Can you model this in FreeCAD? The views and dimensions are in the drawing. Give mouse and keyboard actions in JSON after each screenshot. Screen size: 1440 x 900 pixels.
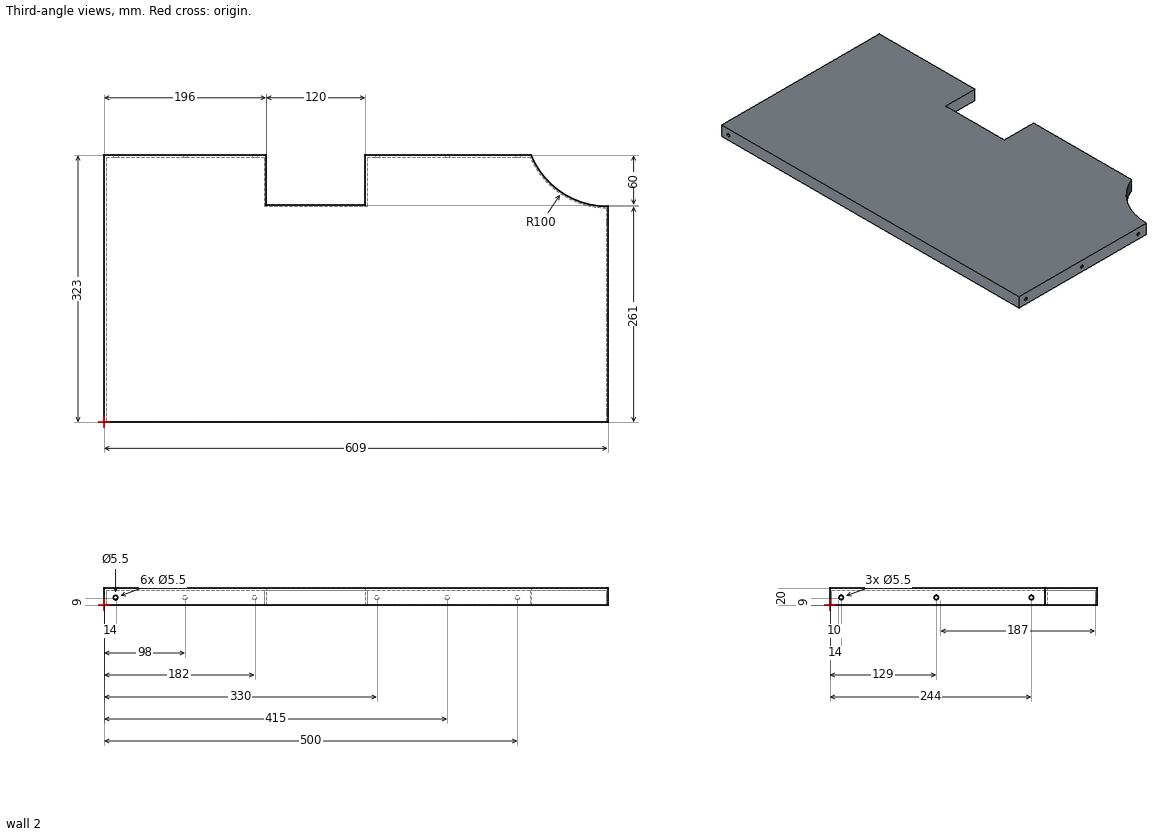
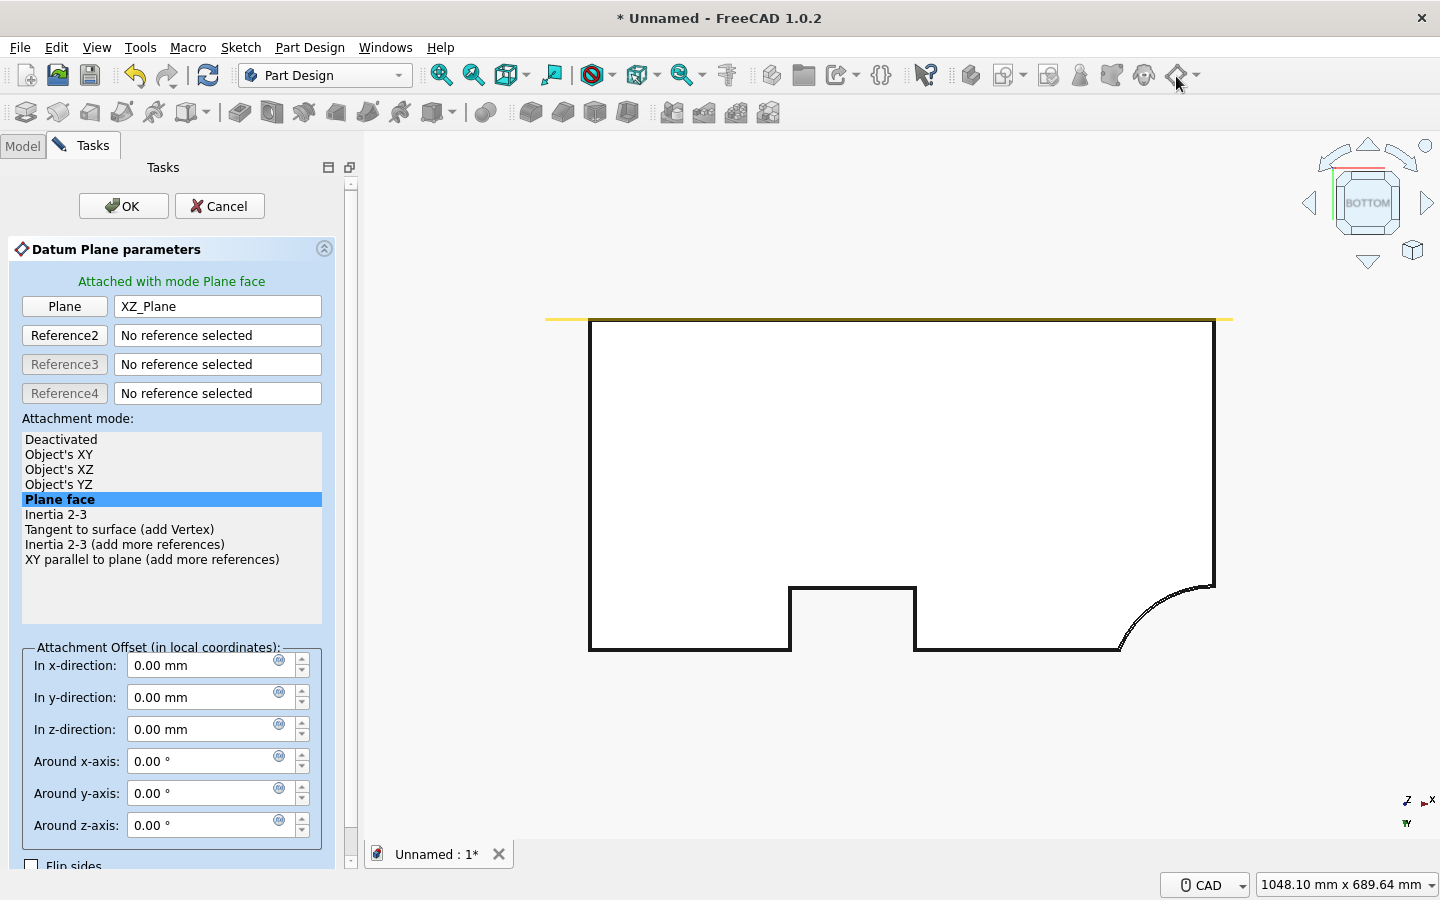
{"action": "triple_click", "coordinate": [210, 729]}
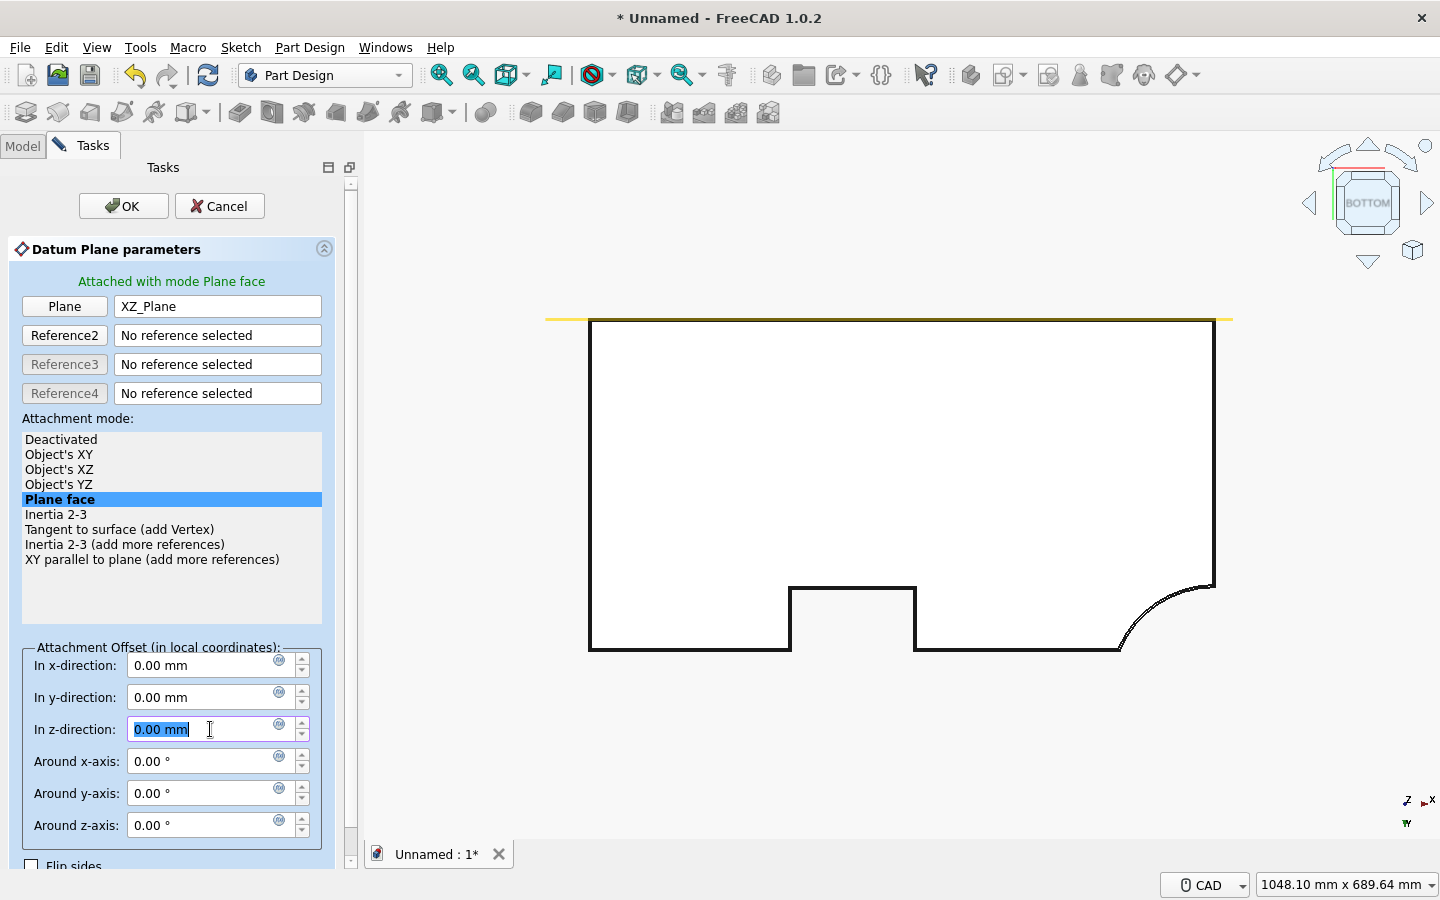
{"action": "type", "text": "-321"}
{"action": "key", "text": "Tab"}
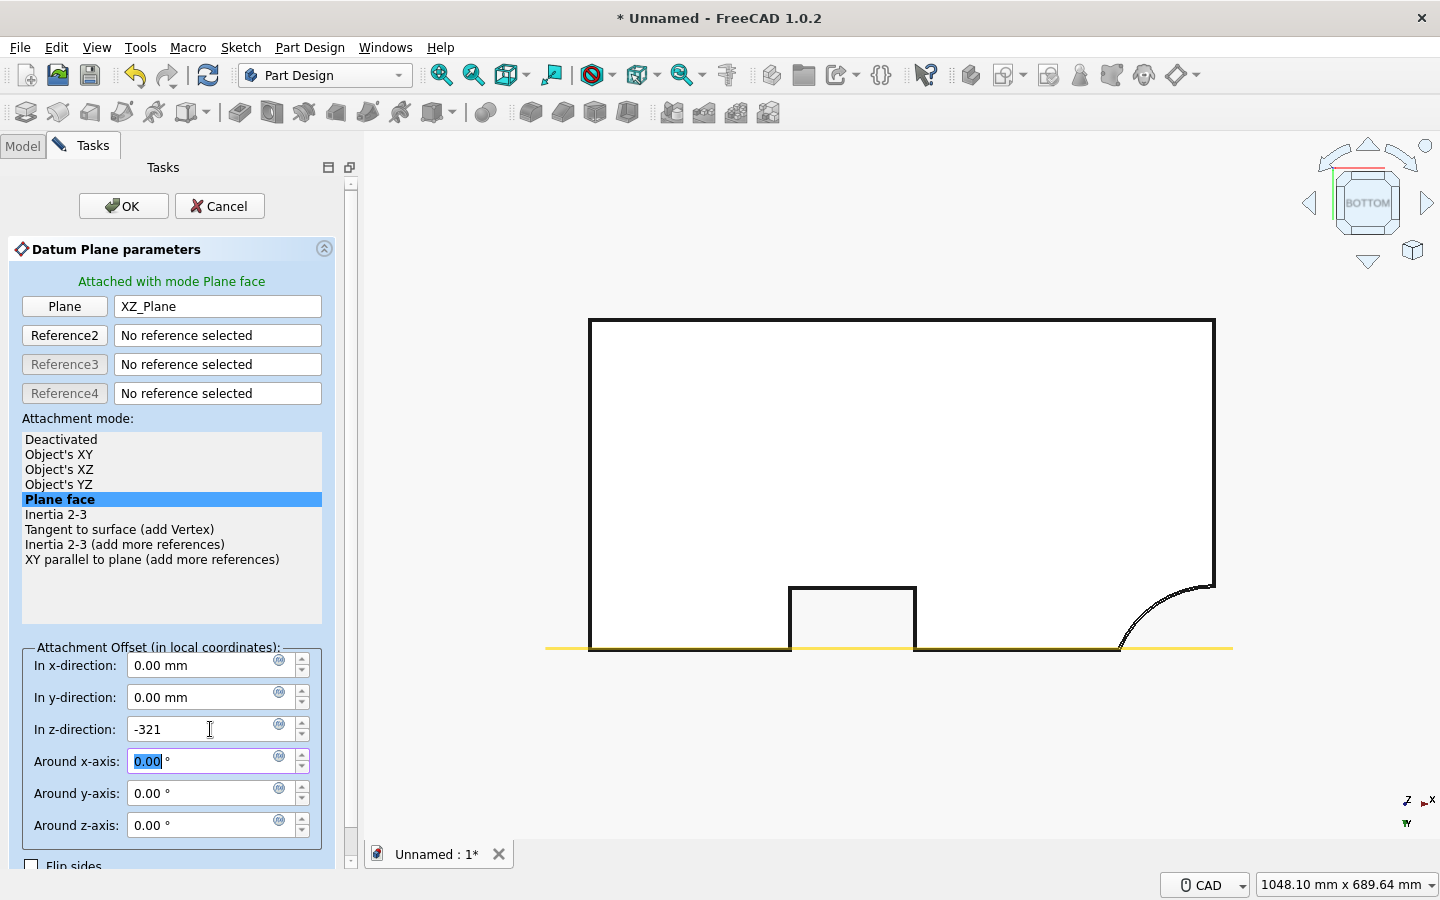
{"action": "left_click", "coordinate": [124, 206]}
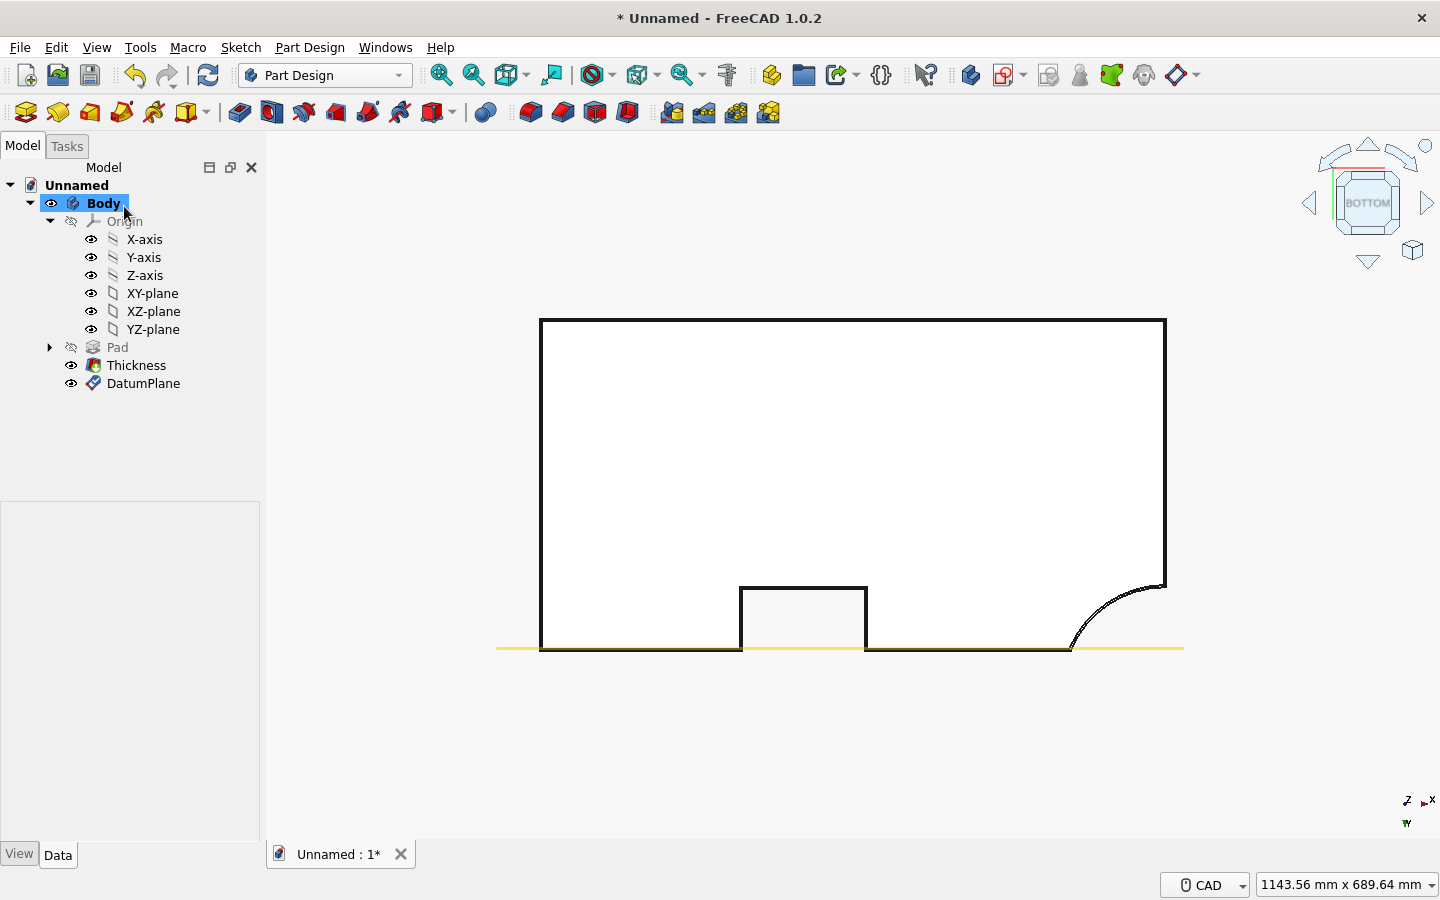
{"action": "left_click", "coordinate": [116, 383]}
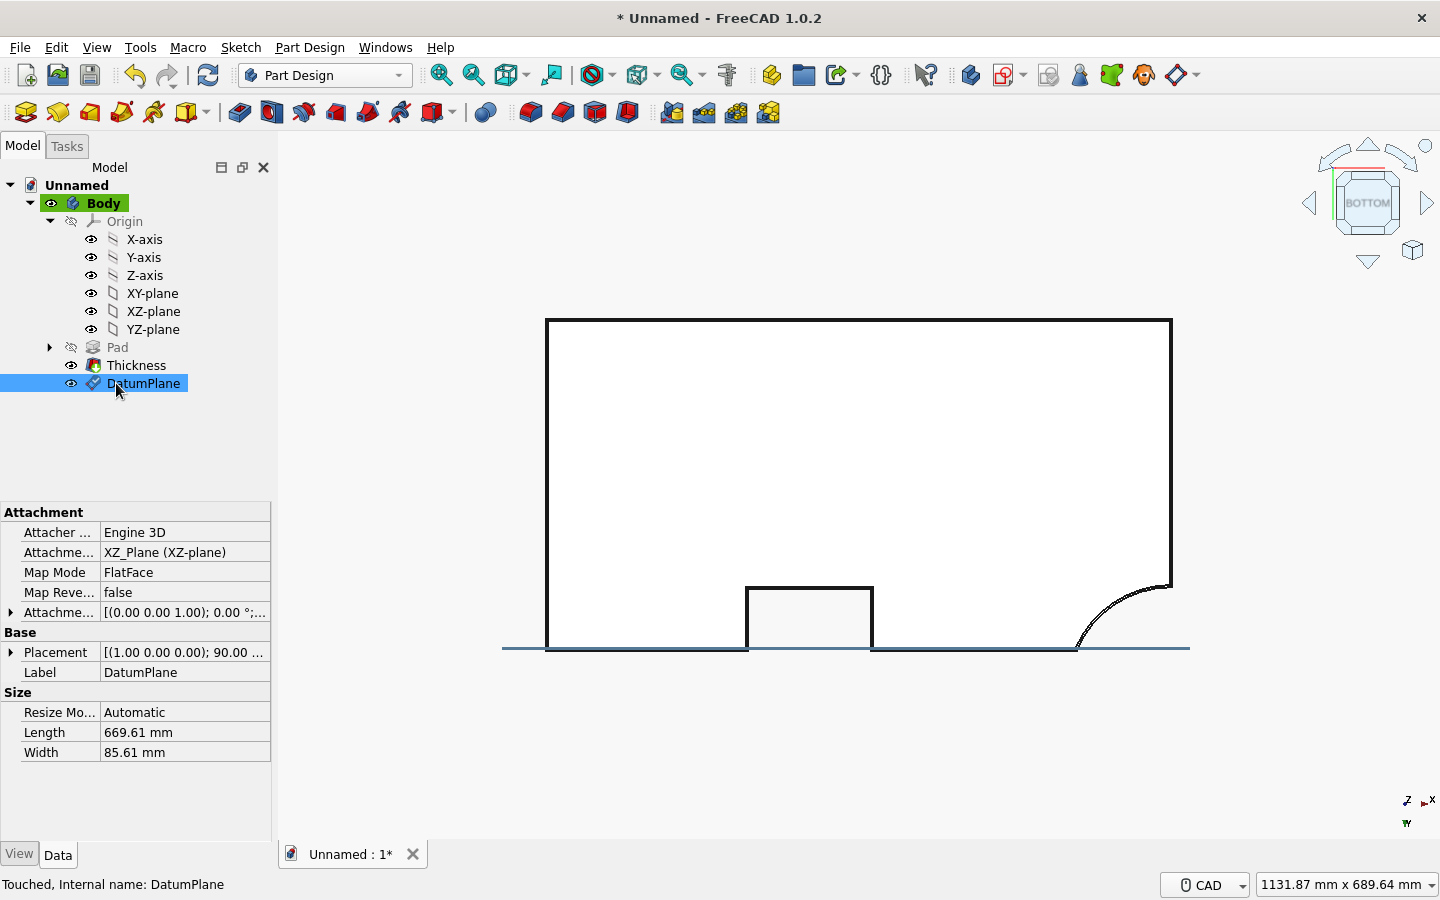
{"action": "left_click", "coordinate": [1004, 76]}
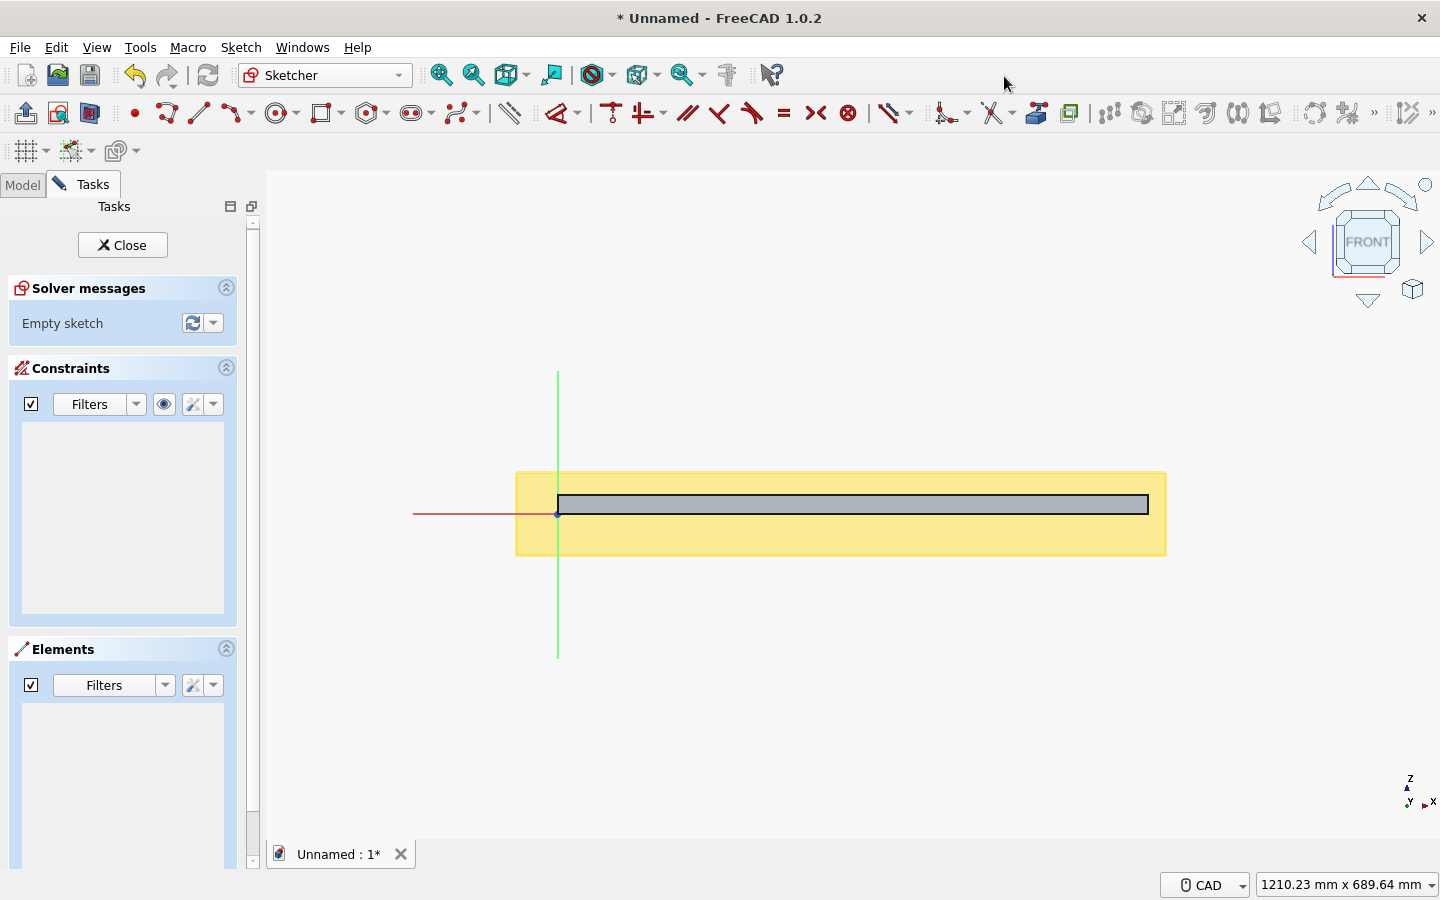
{"action": "key", "text": "q s"}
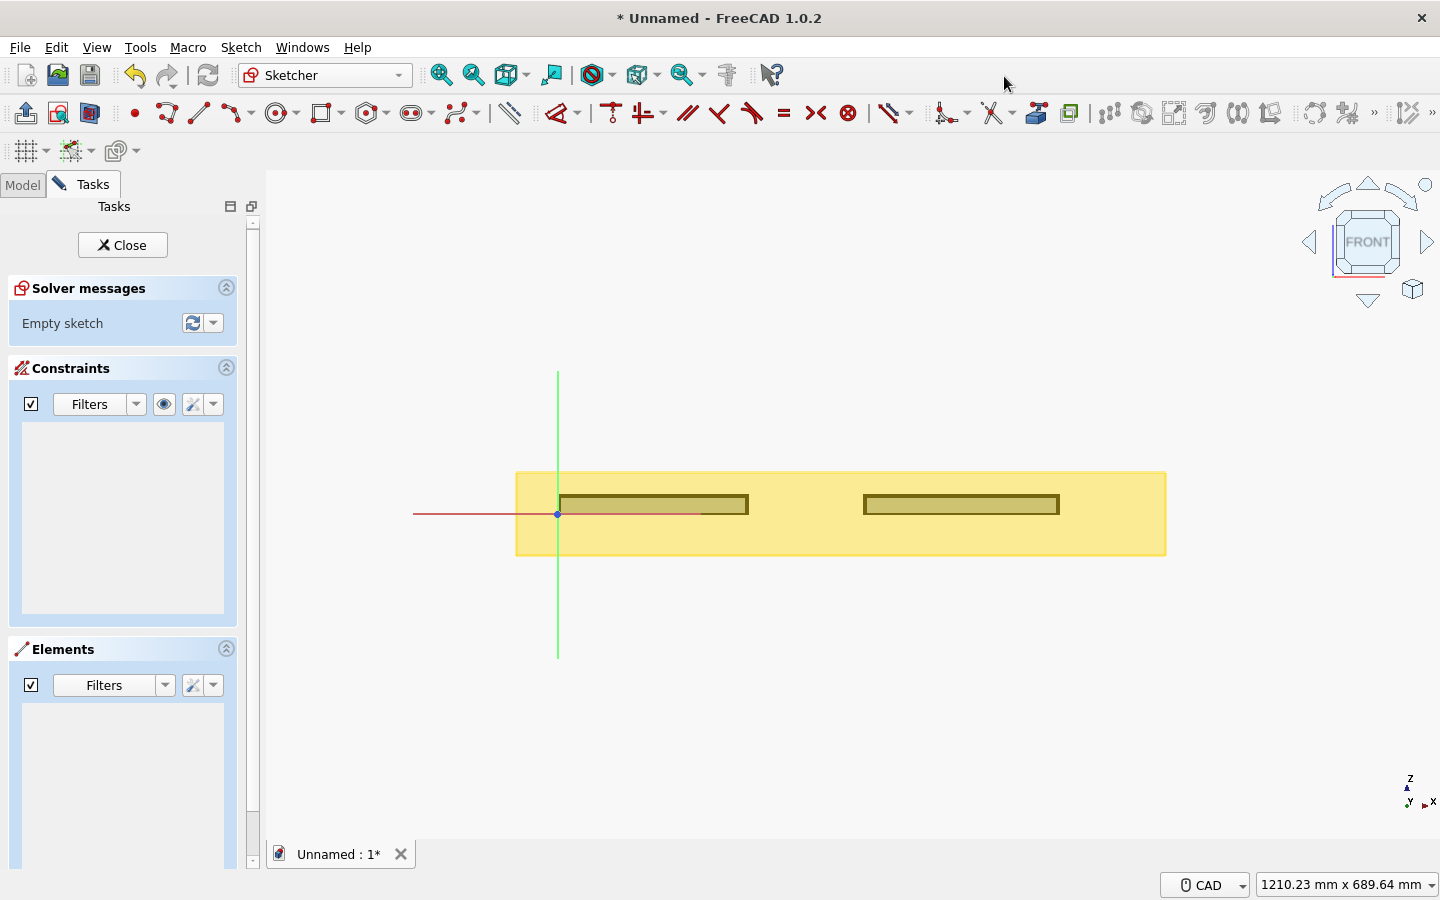
{"action": "scroll", "coordinate": [836, 517], "scroll_direction": "up", "scroll_amount": 2}